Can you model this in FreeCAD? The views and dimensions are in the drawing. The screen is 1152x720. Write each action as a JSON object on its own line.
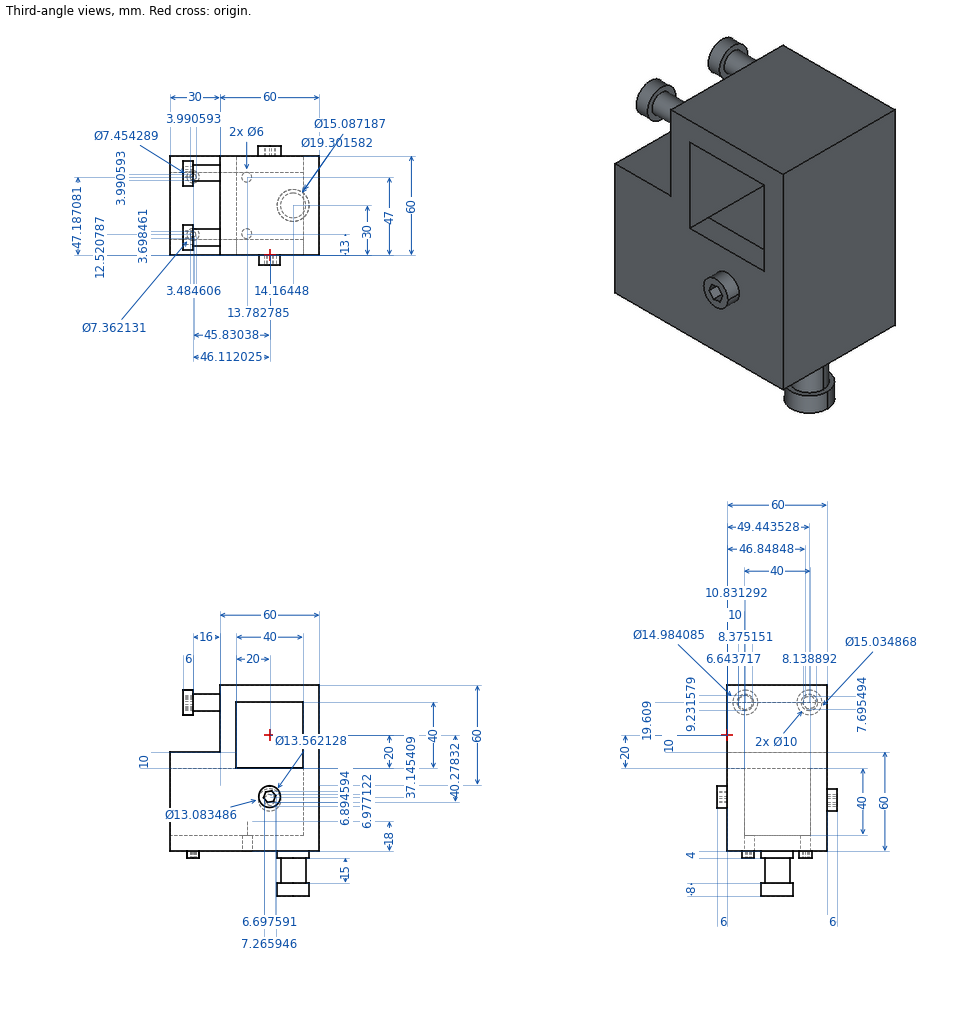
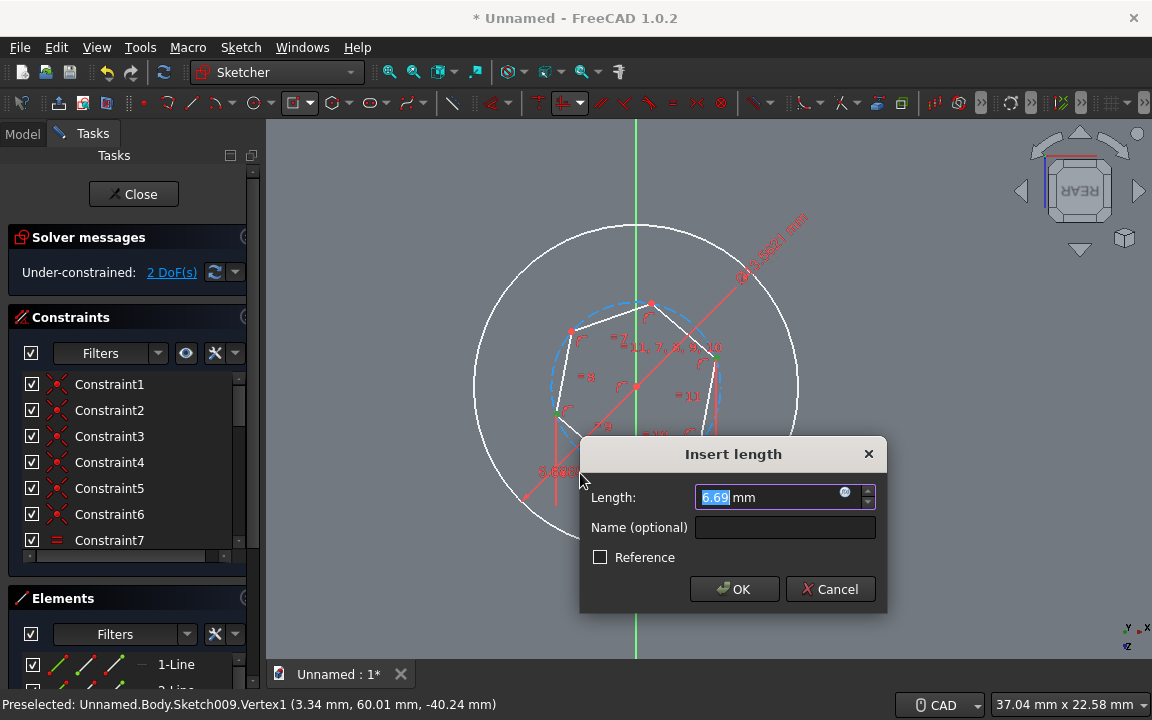
{"action": "type", "text": "6.697591"}
{"action": "key", "text": "Return"}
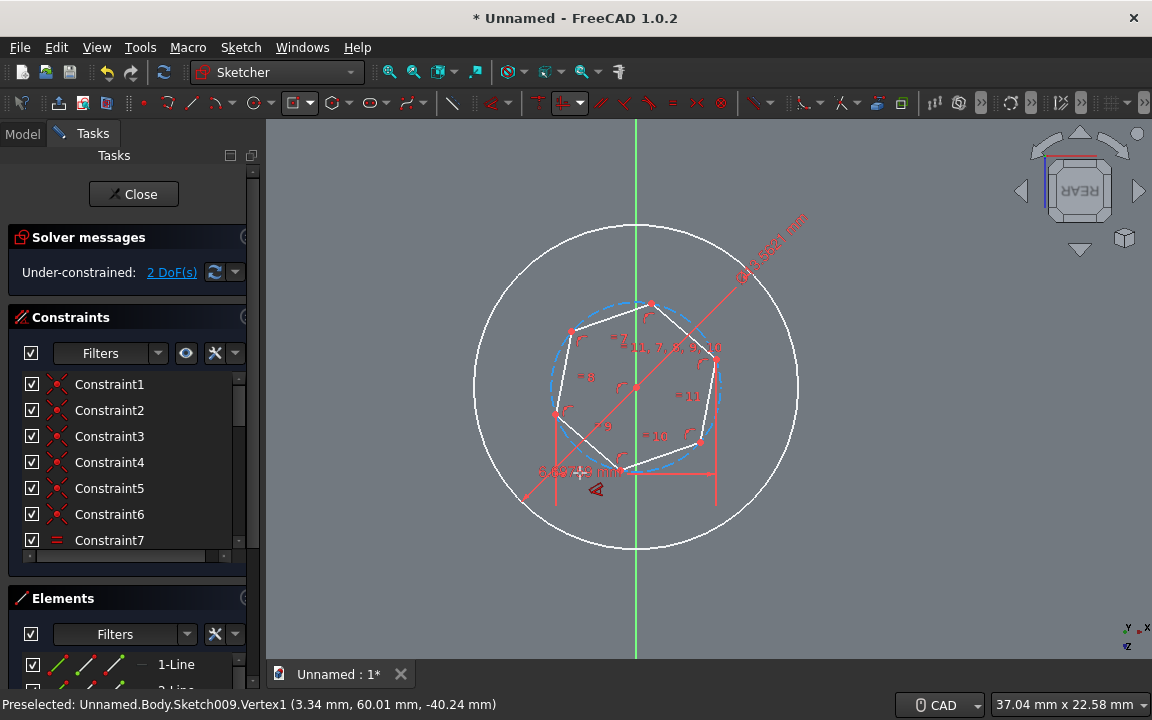
{"action": "left_click", "coordinate": [620, 470]}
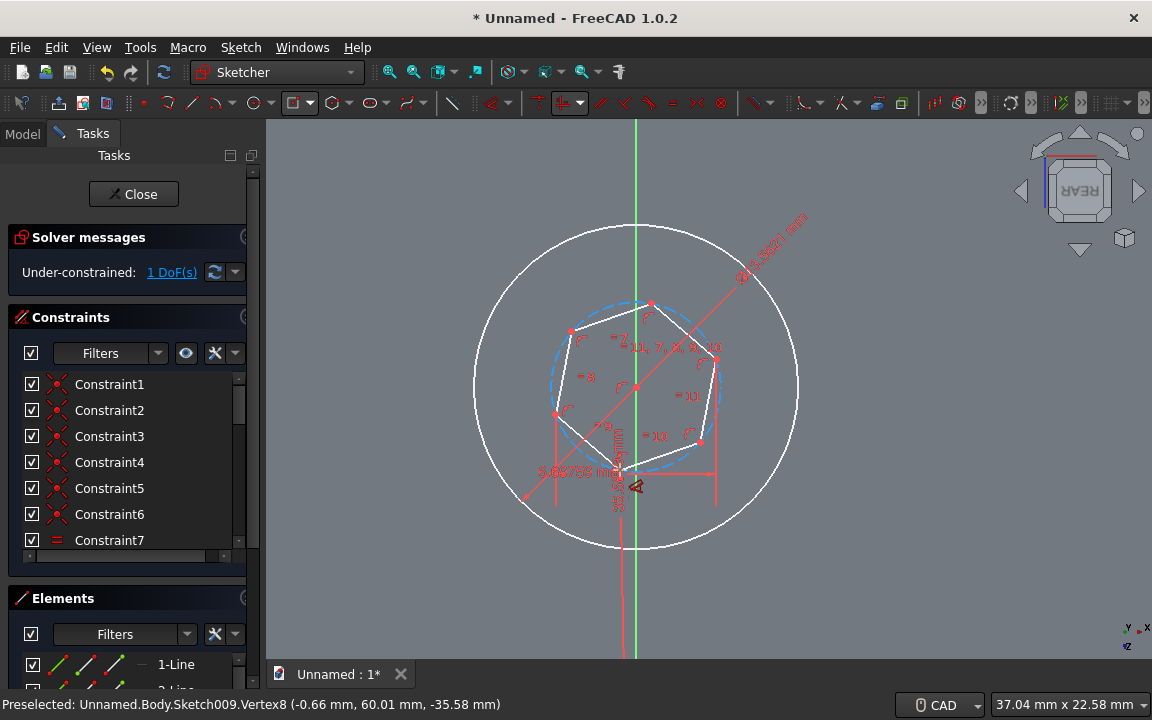
{"action": "left_click", "coordinate": [652, 304]}
{"action": "left_click", "coordinate": [686, 387]}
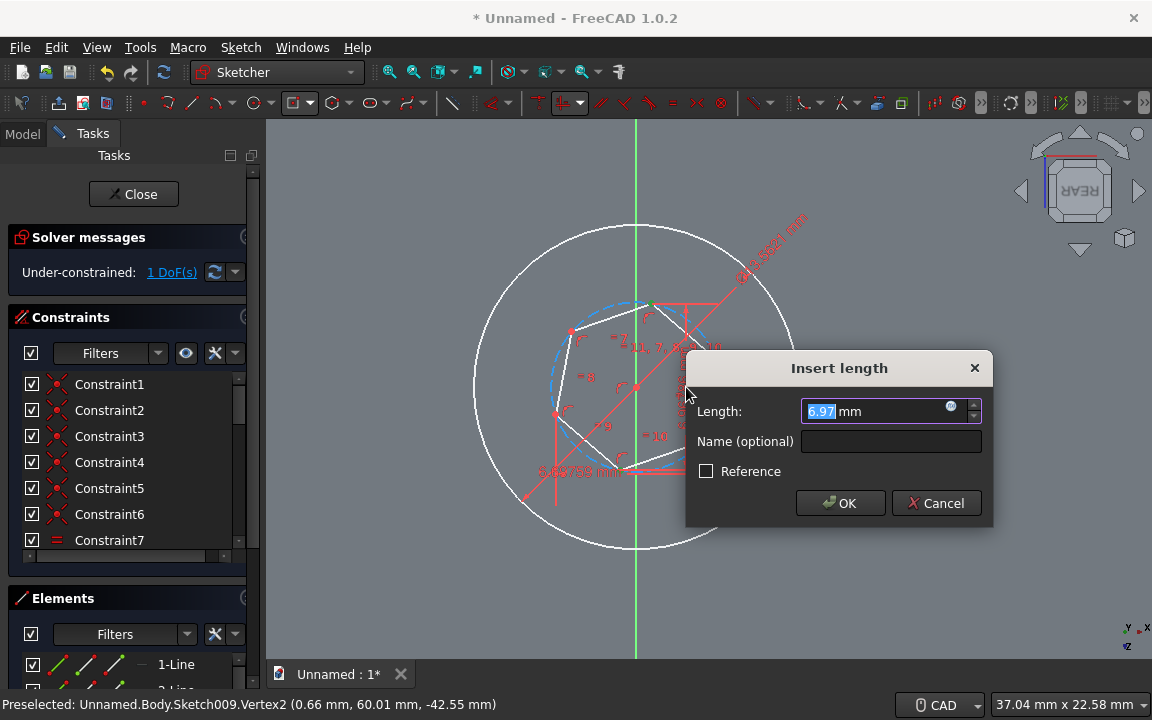
{"action": "type", "text": "6.977122"}
{"action": "key", "text": "Return"}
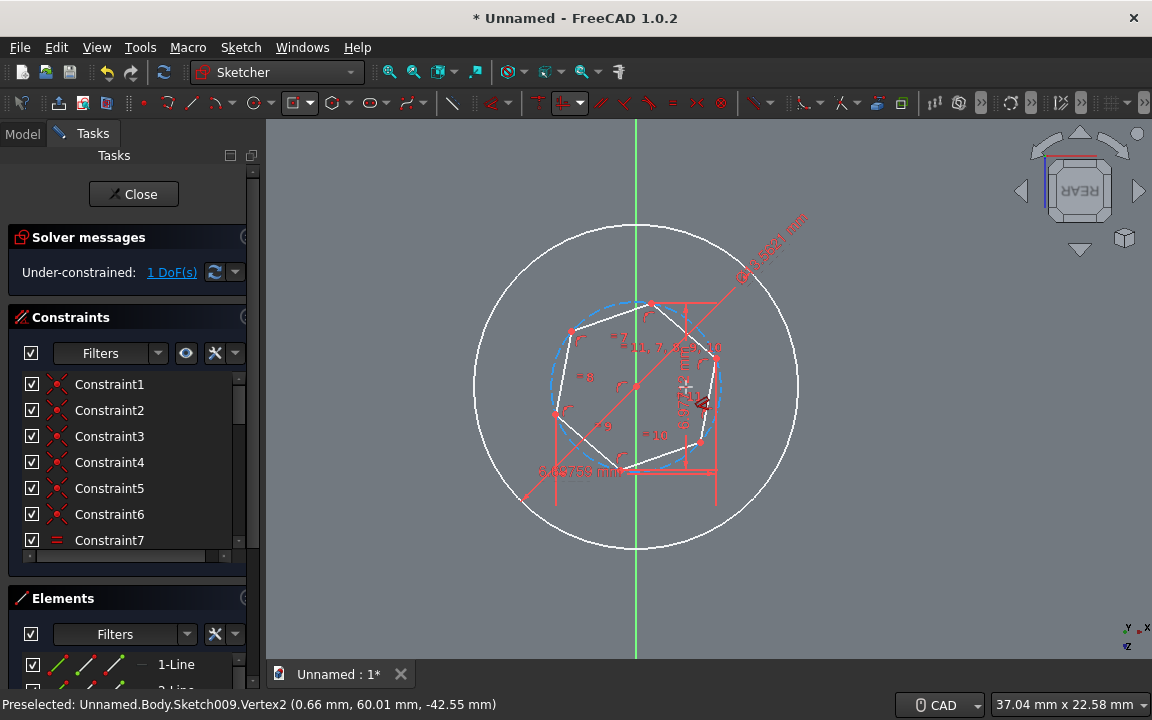
{"action": "left_click", "coordinate": [716, 359]}
{"action": "left_click", "coordinate": [750, 432]}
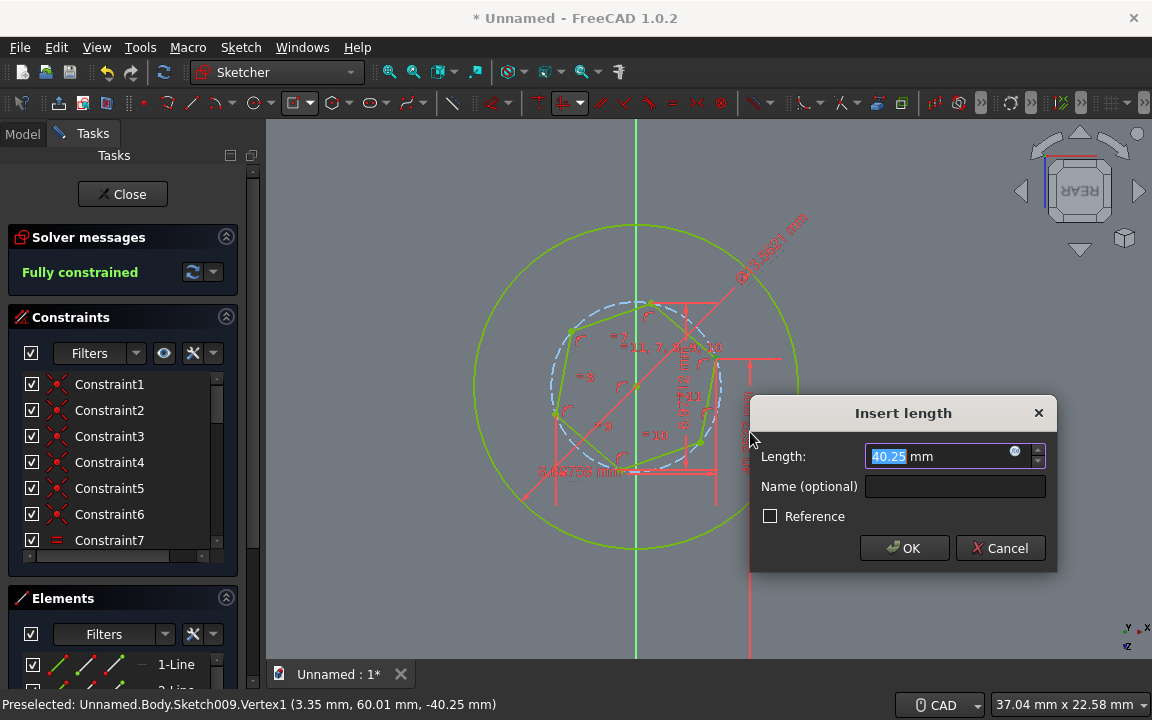
{"action": "type", "text": "40.27832"}
{"action": "key", "text": "Return"}
{"action": "key", "text": "Escape"}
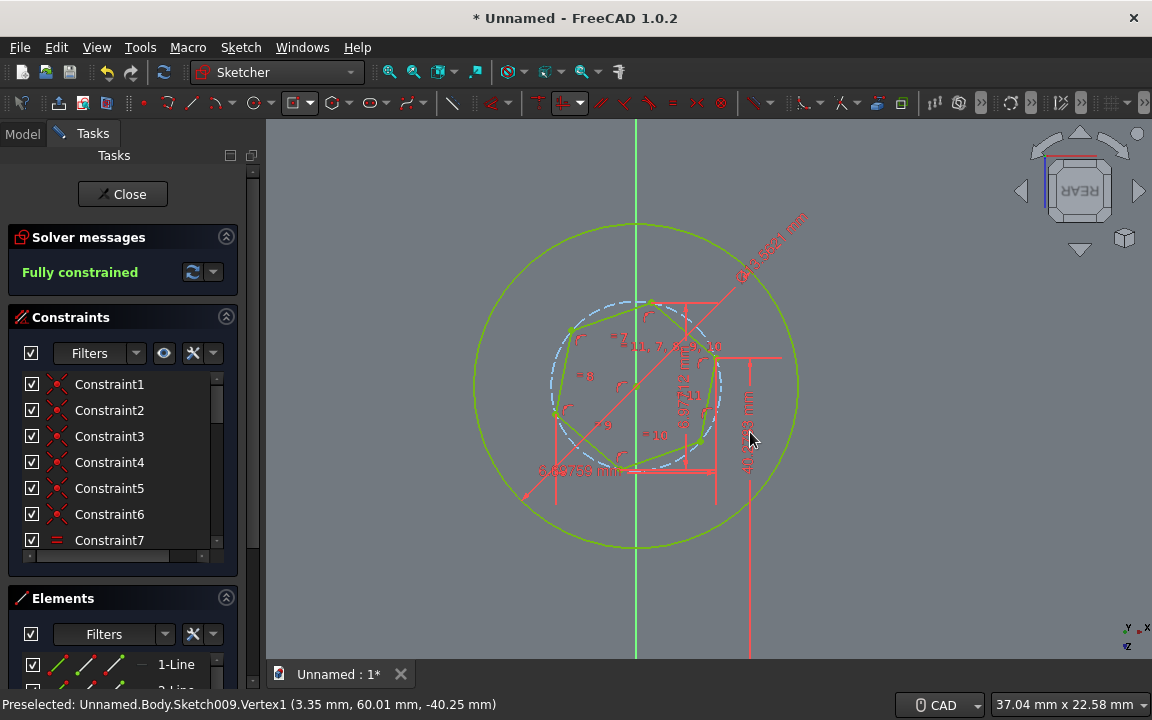
{"action": "left_click", "coordinate": [123, 194]}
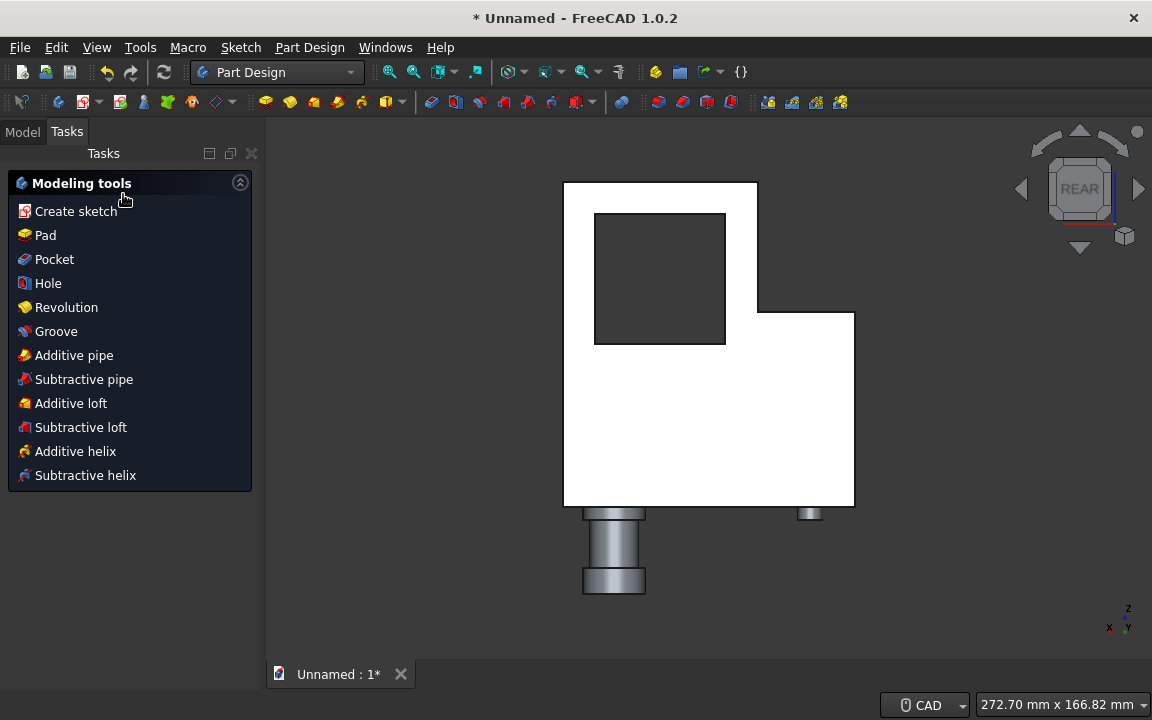
{"action": "left_click", "coordinate": [266, 102]}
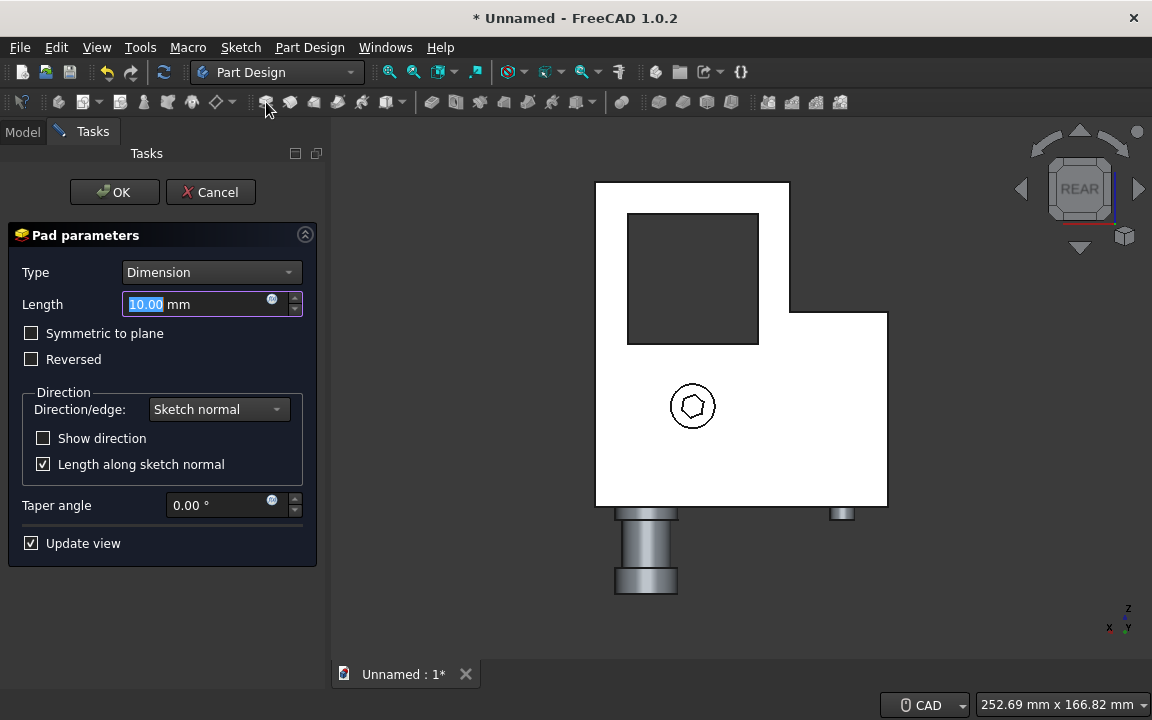
{"action": "type", "text": "6"}
{"action": "key", "text": "Tab"}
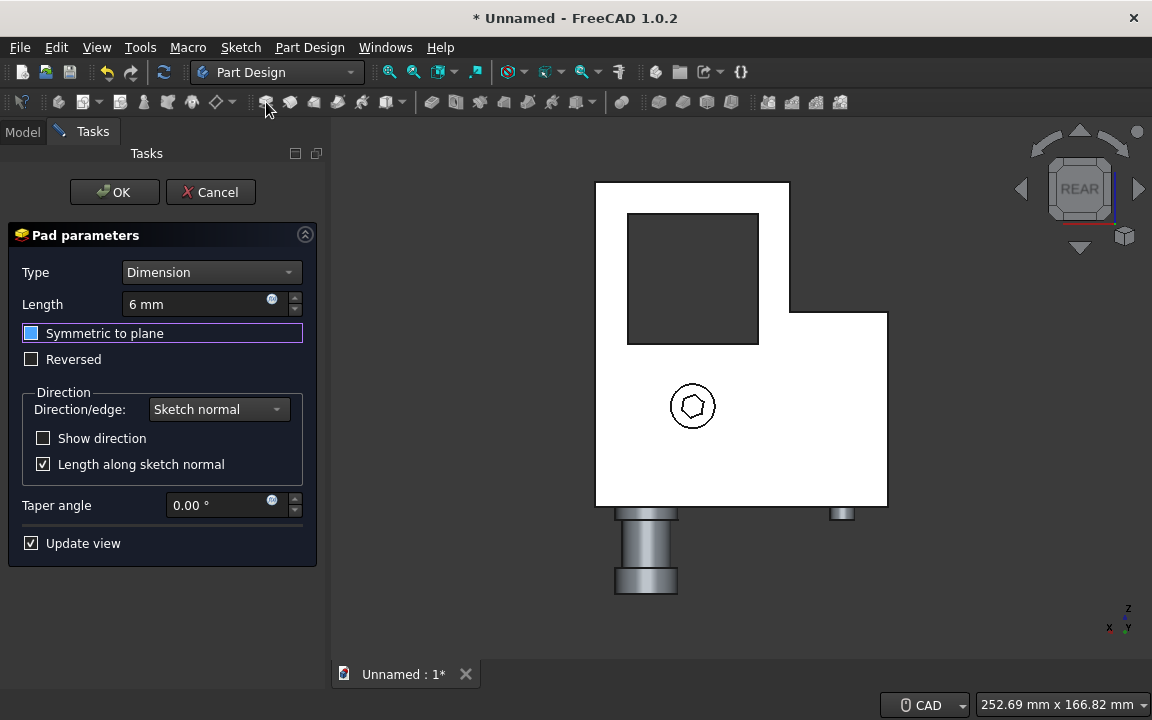
{"action": "left_click", "coordinate": [115, 192]}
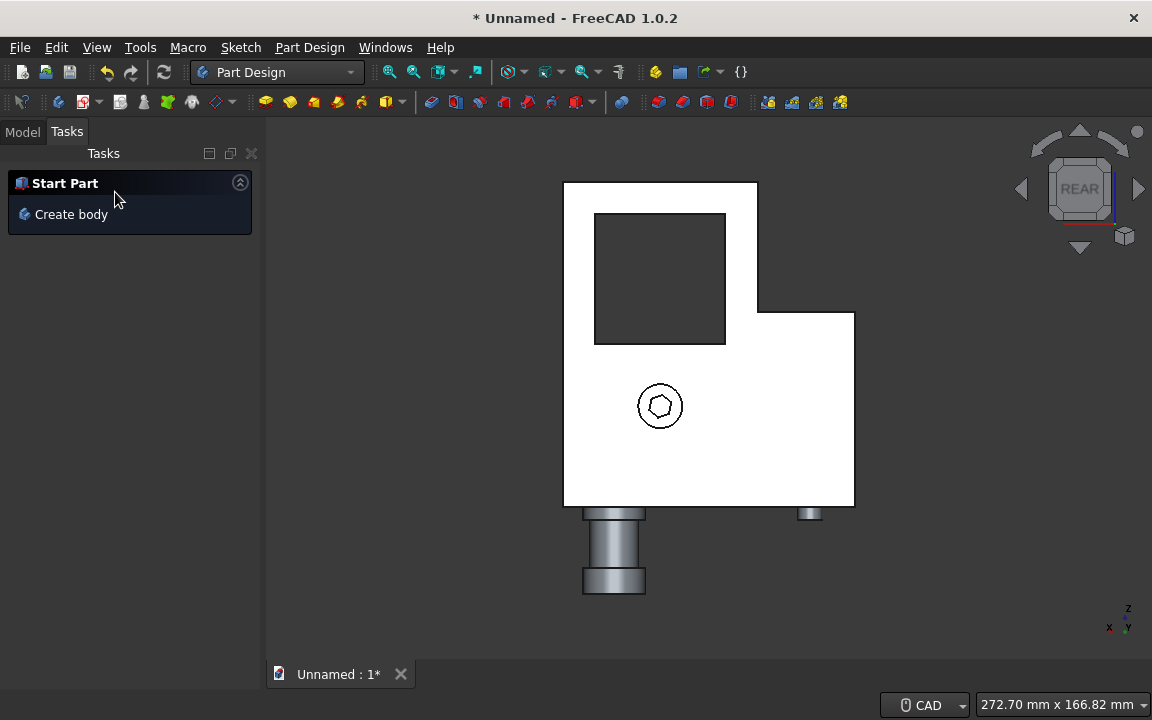
{"action": "key", "text": "0"}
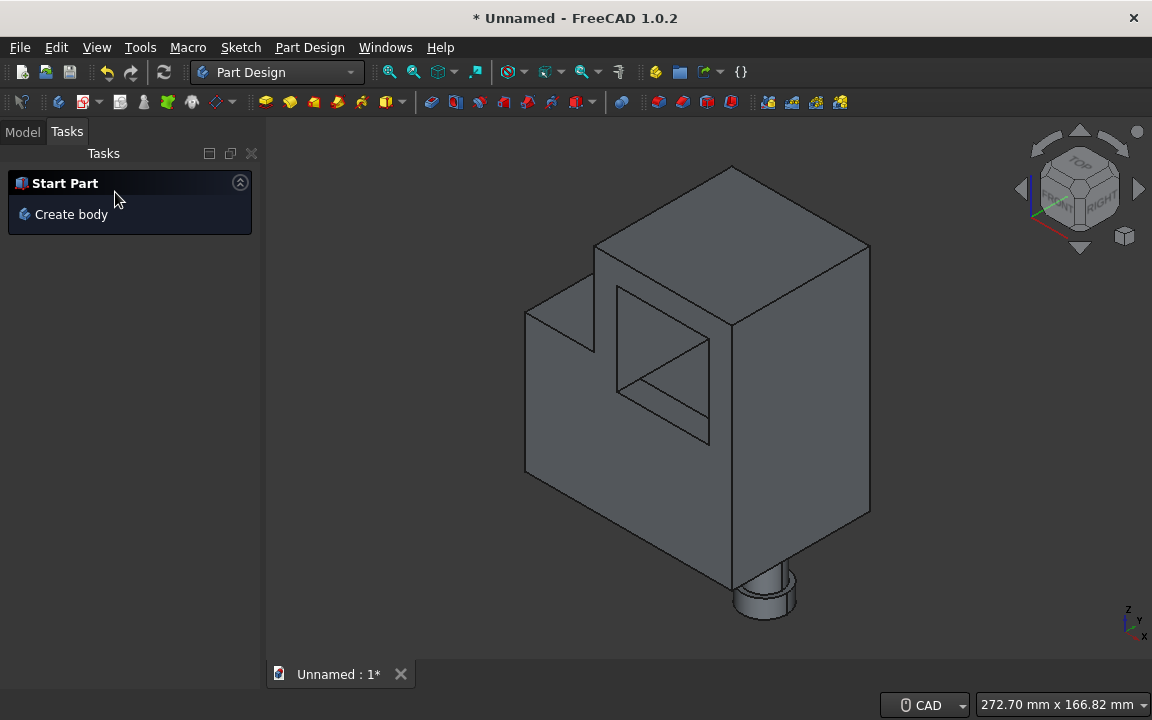
{"action": "left_click", "coordinate": [390, 72]}